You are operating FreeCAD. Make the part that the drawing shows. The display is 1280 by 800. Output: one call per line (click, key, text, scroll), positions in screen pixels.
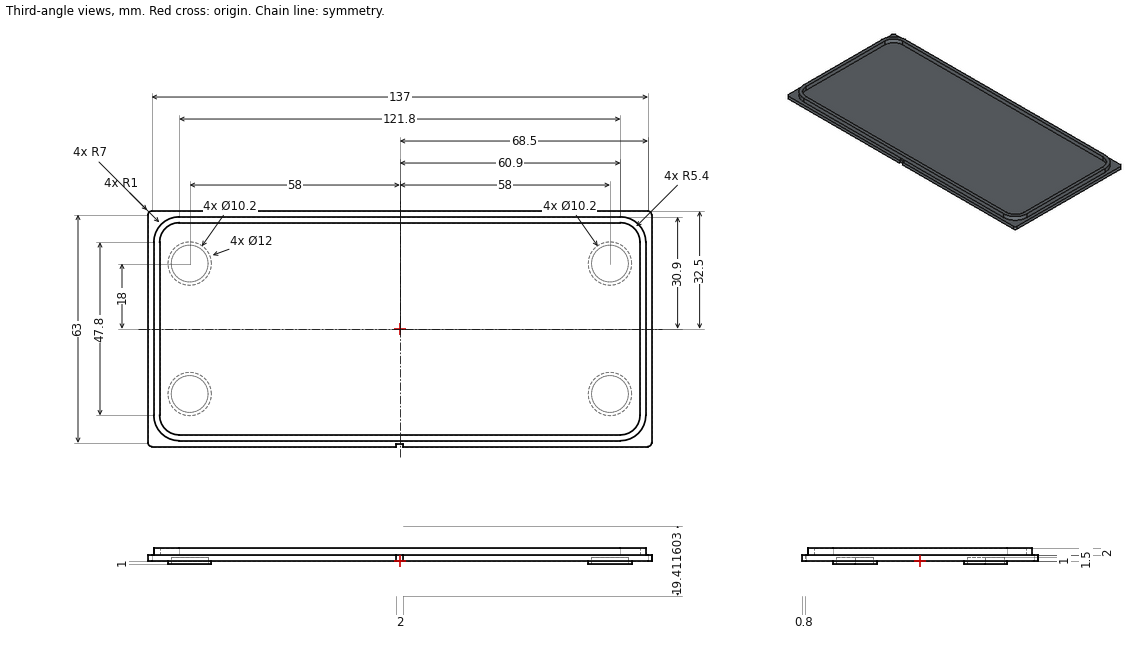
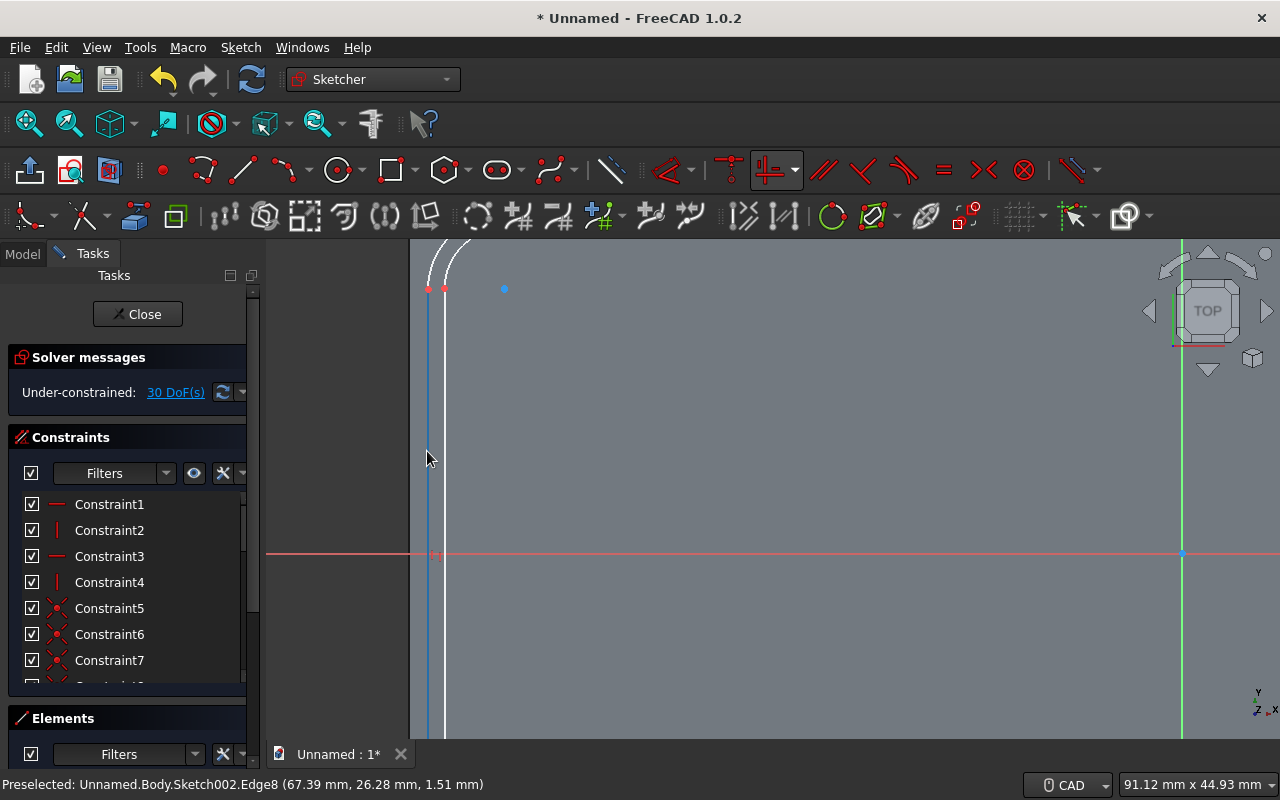
click(428, 450)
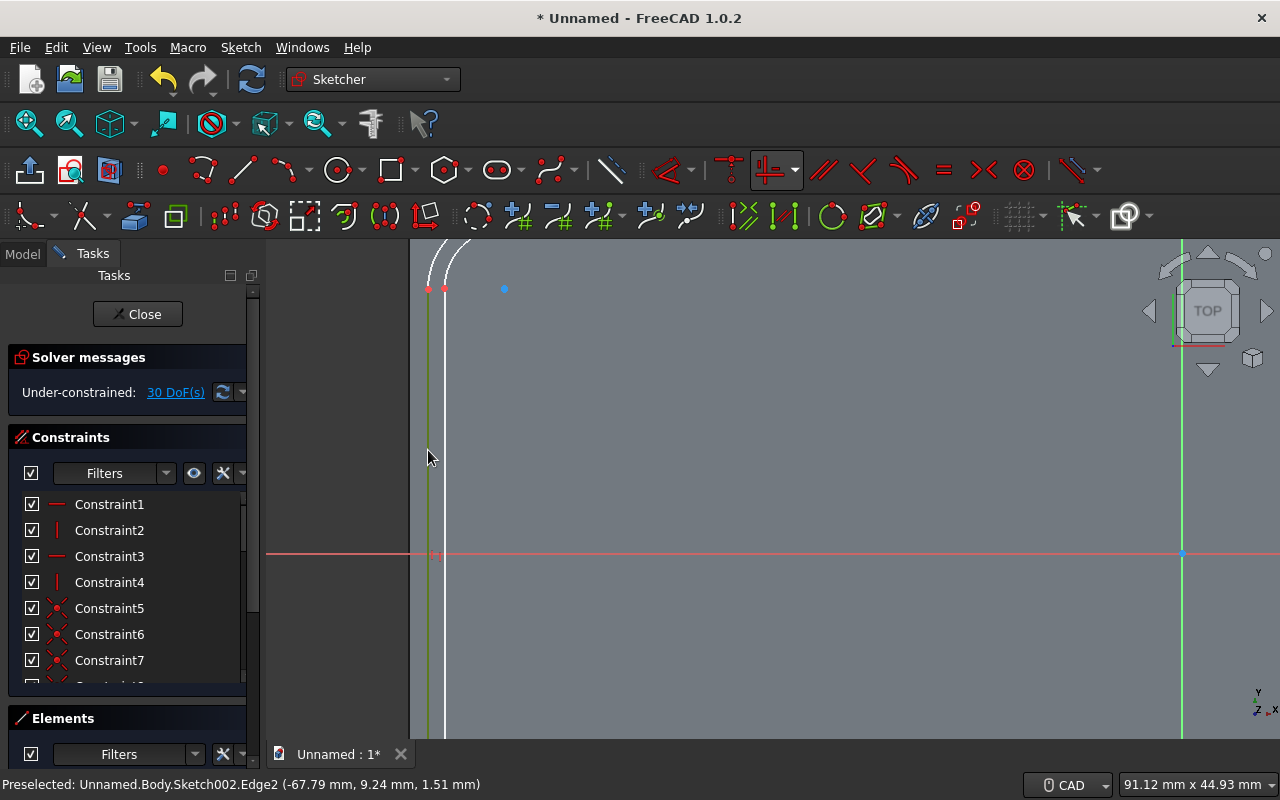
scroll(426, 451, down, 5)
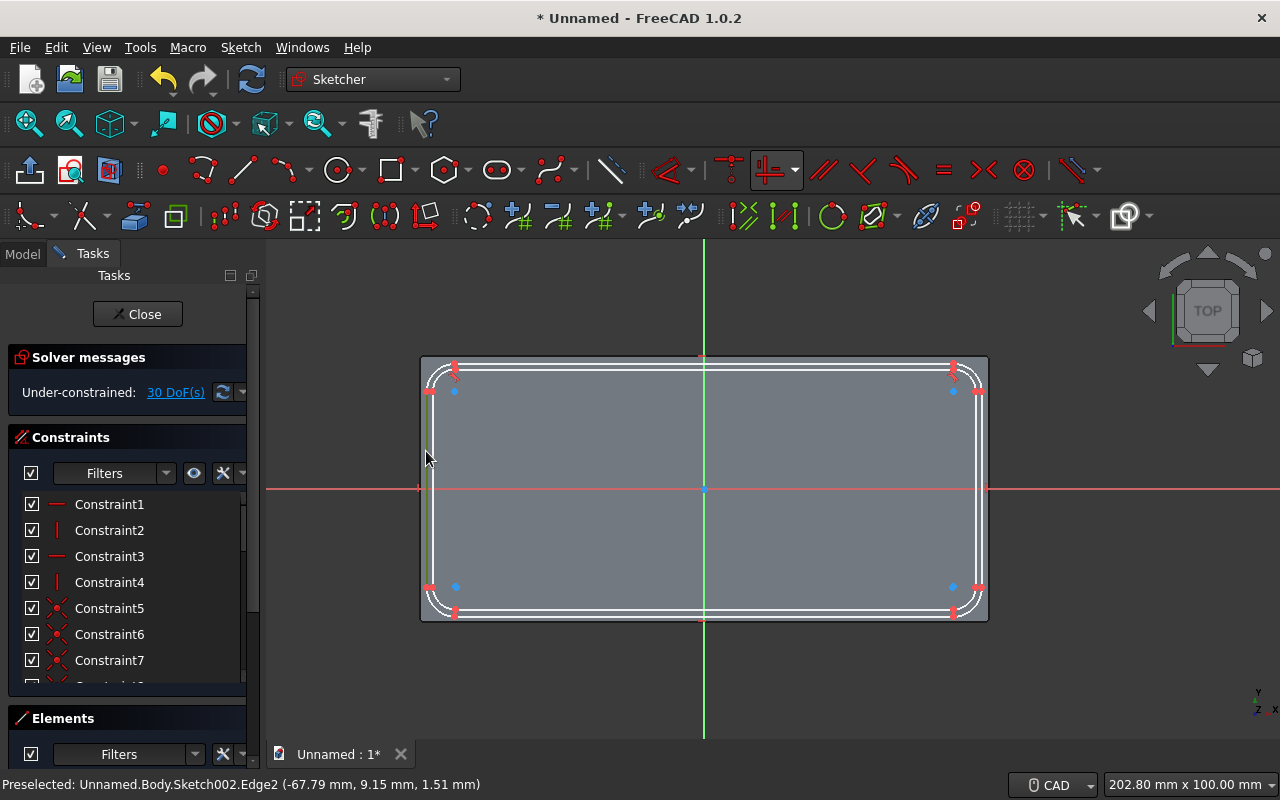
scroll(442, 367, up, 5)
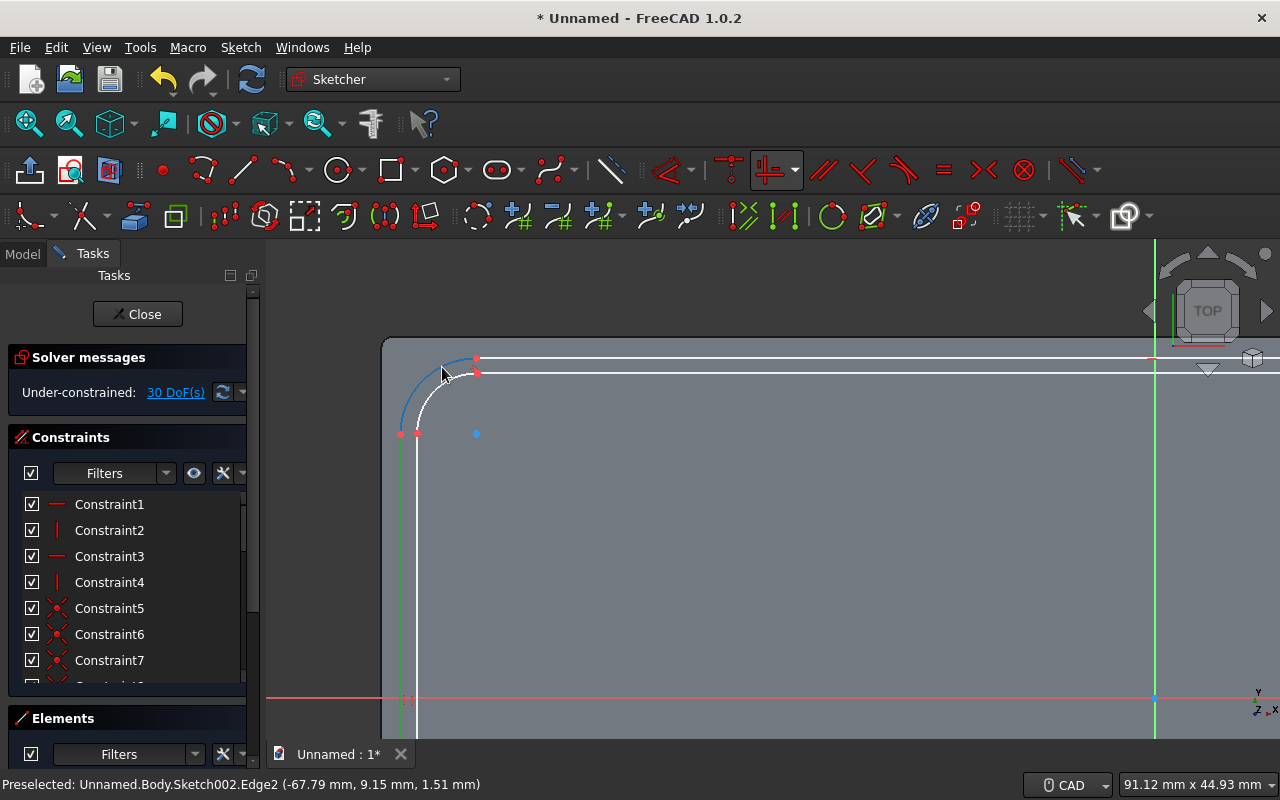
click(442, 367)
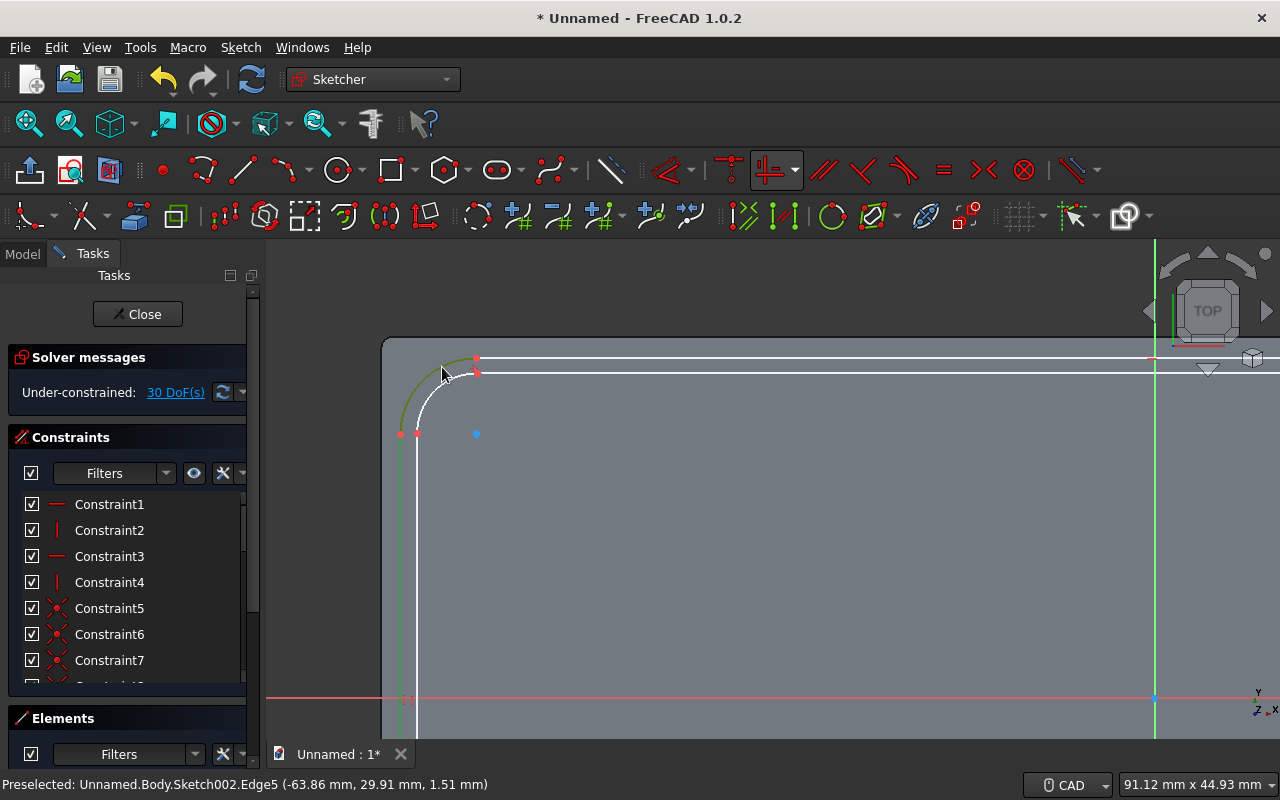
click(904, 170)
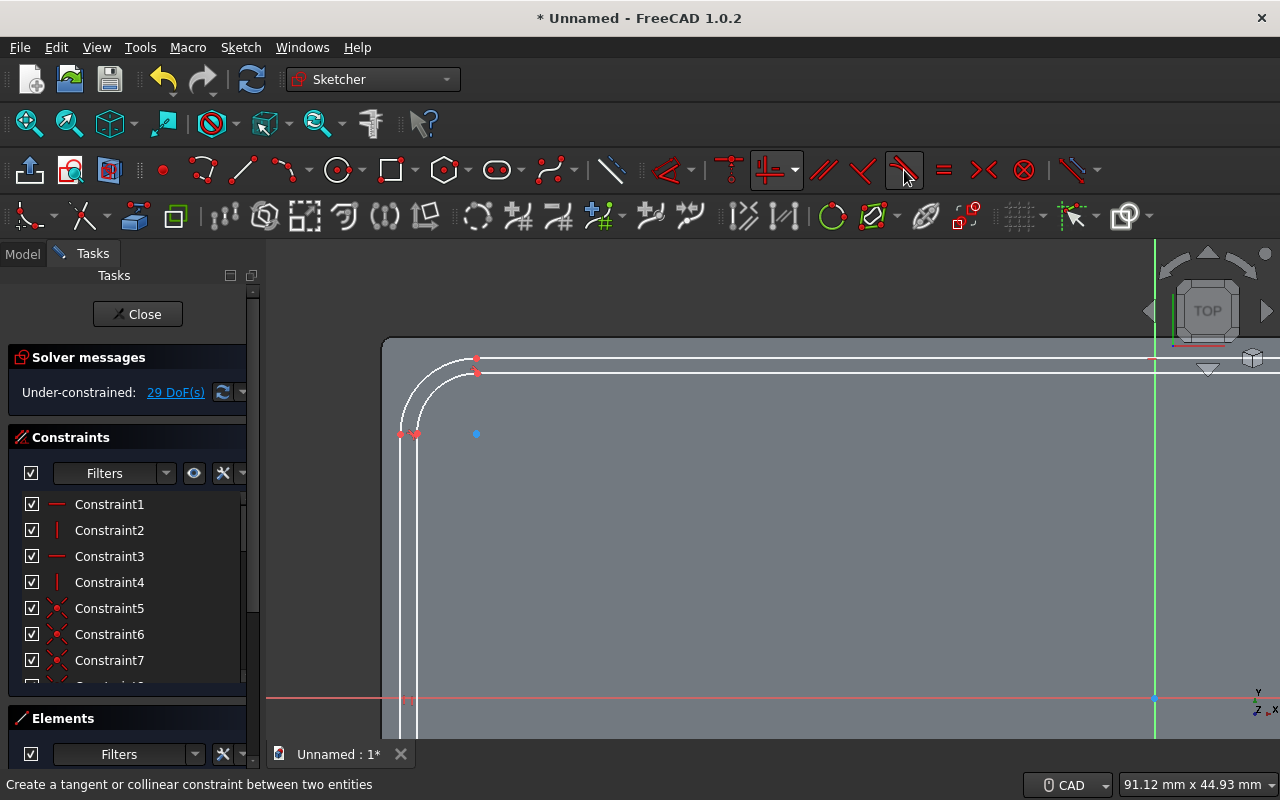
click(400, 594)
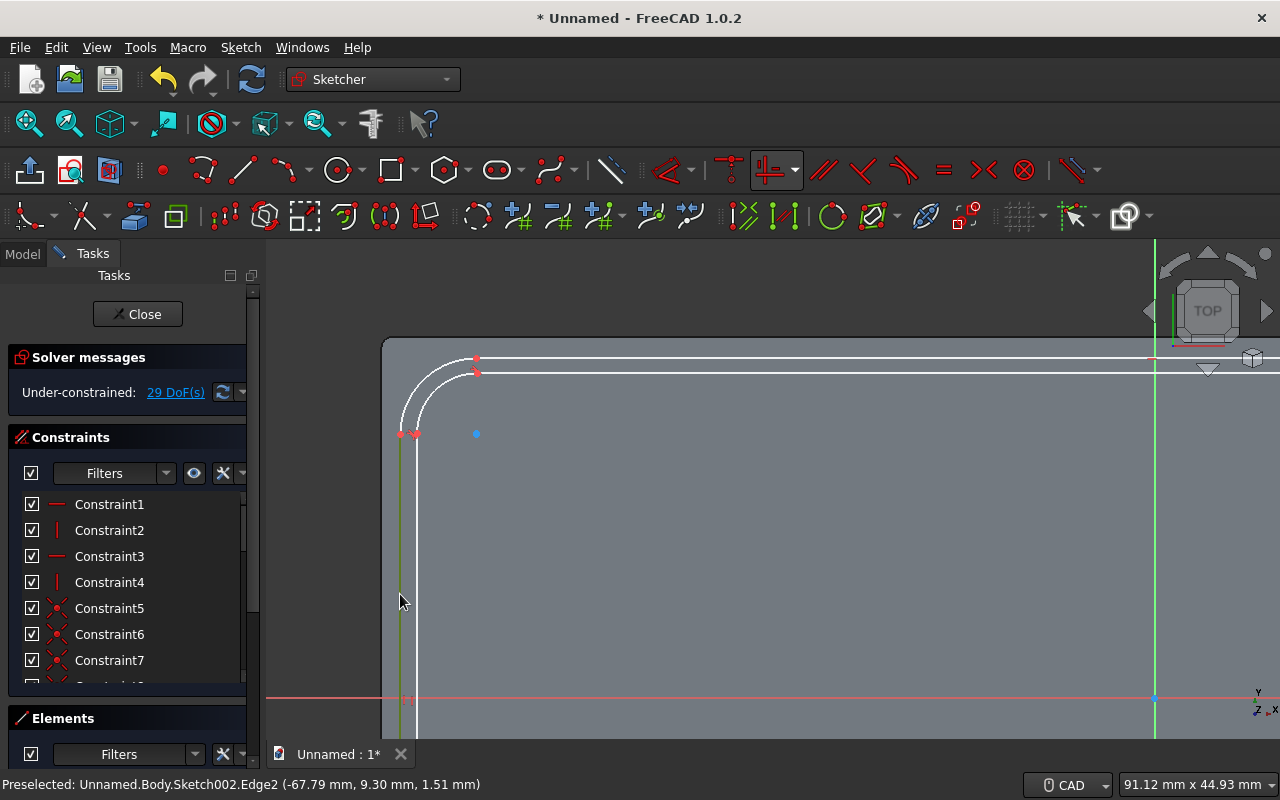
scroll(442, 367, down, 5)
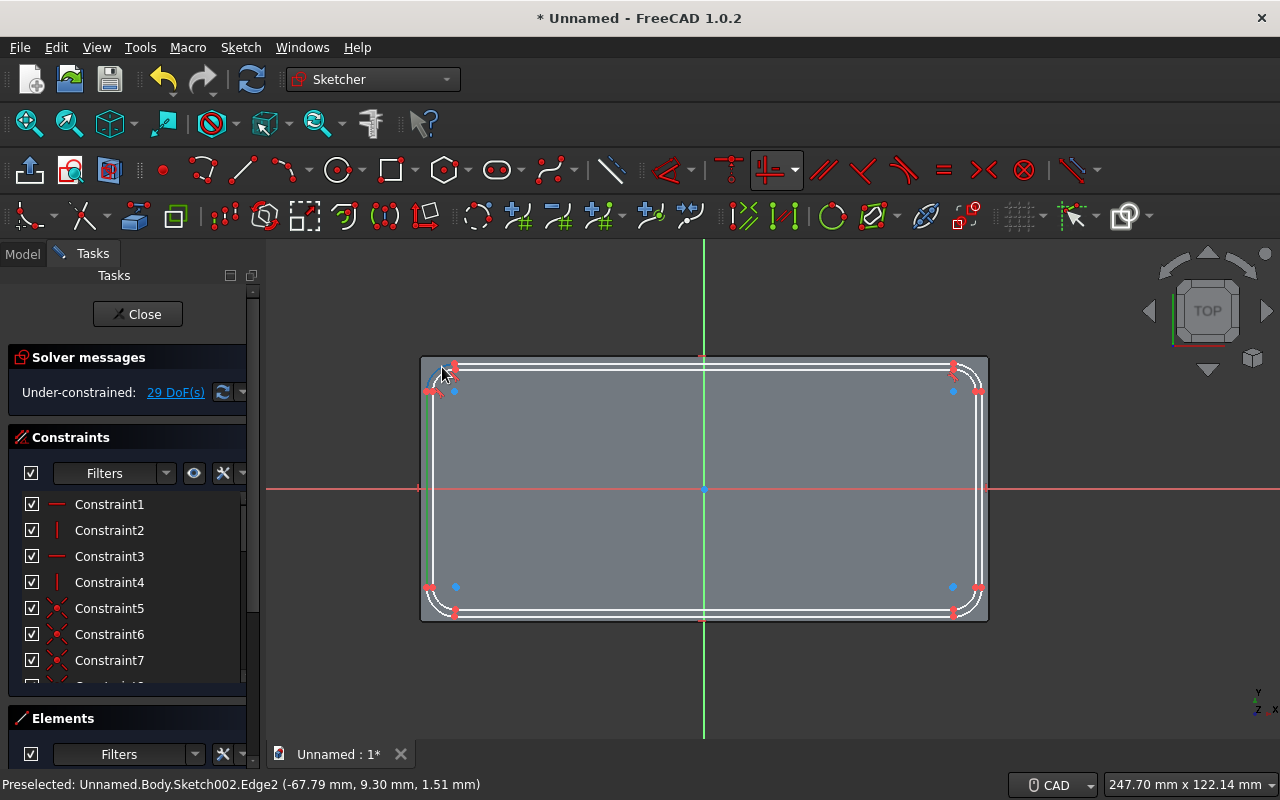
scroll(430, 601, up, 4)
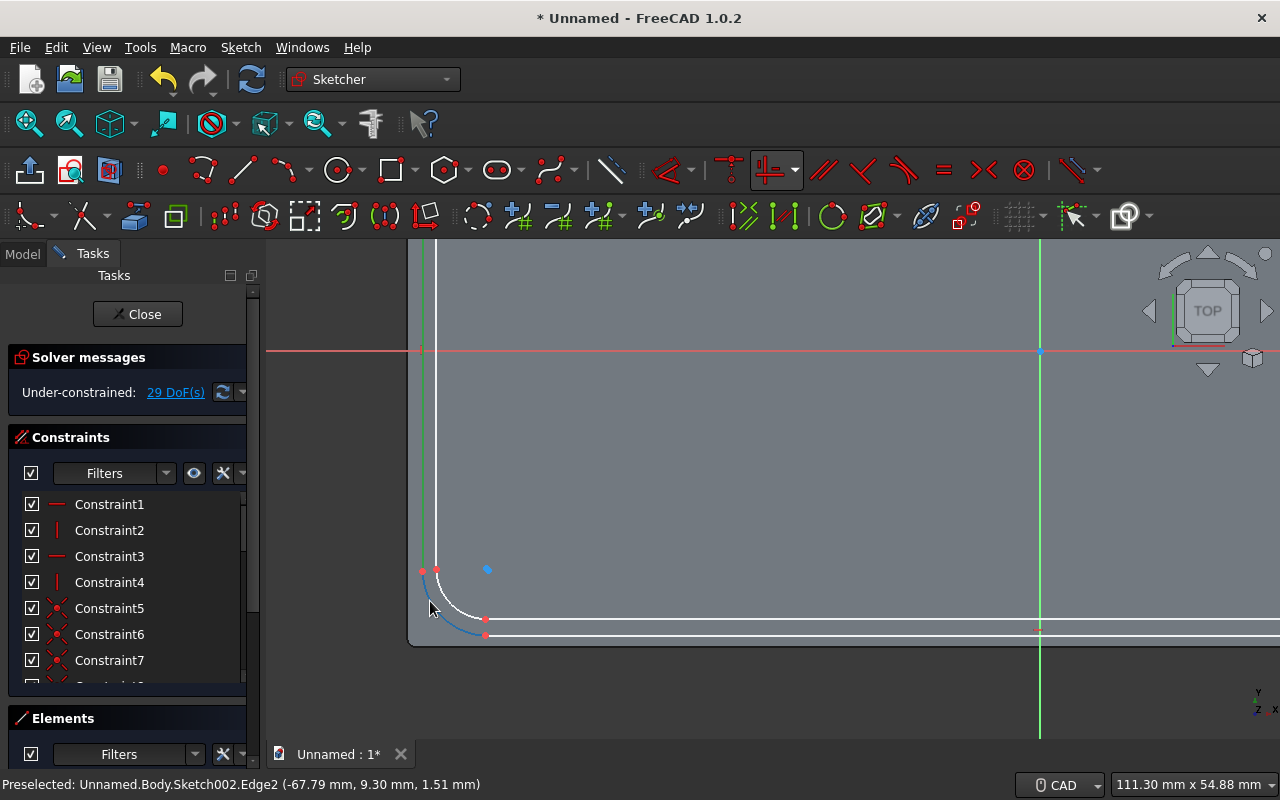
click(430, 600)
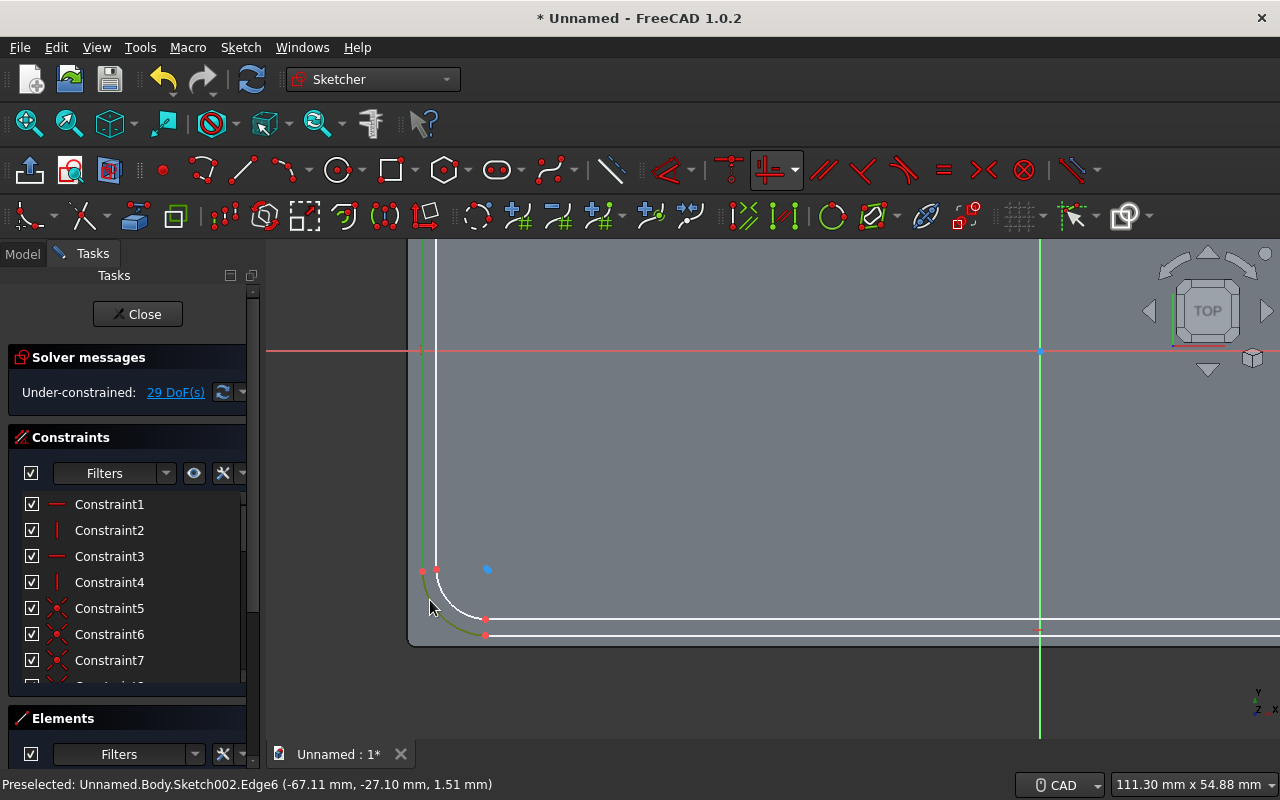
click(904, 170)